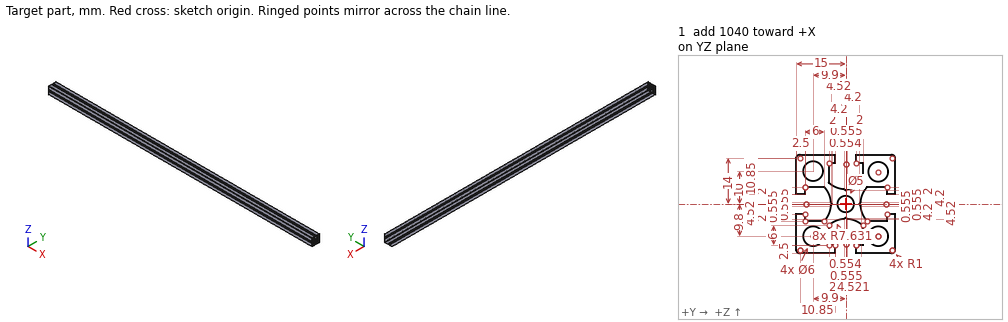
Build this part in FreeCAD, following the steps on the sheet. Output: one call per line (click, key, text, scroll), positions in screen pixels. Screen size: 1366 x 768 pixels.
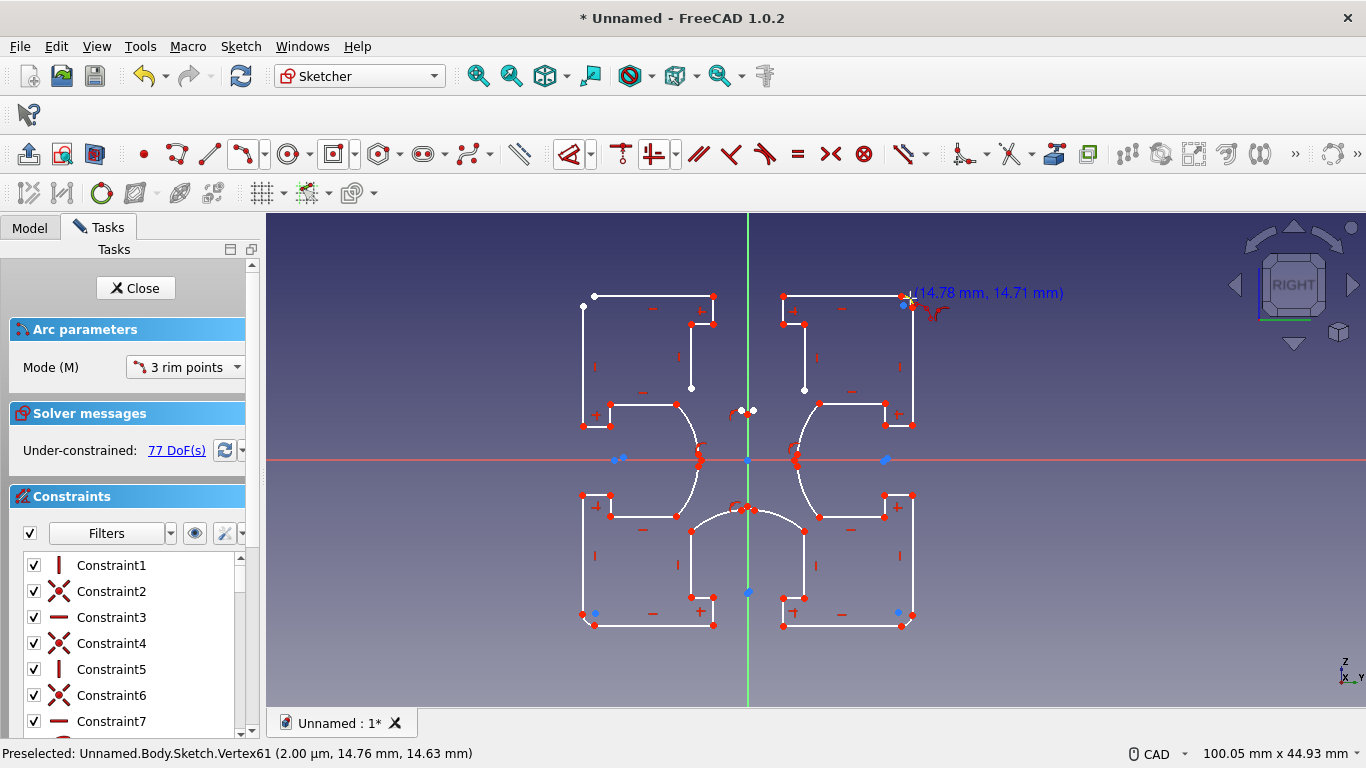
click(805, 390)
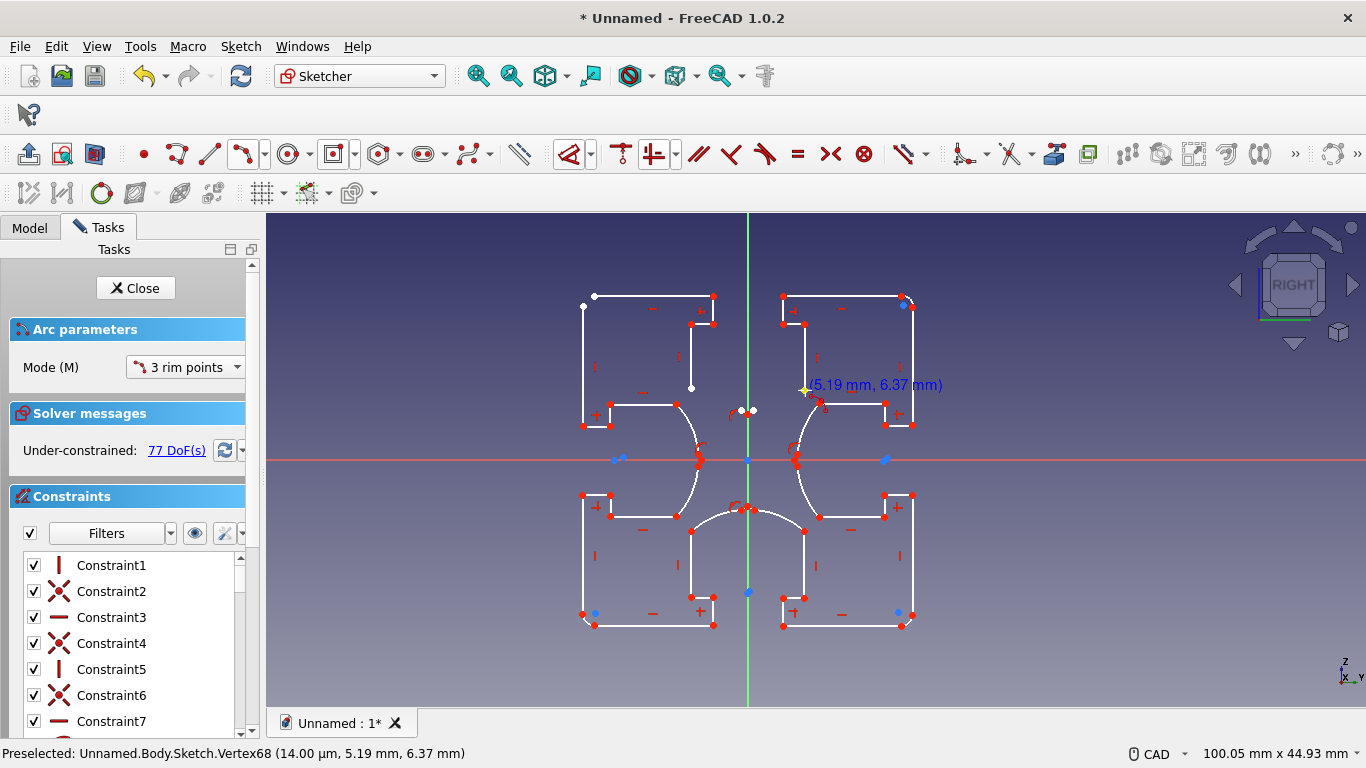
scroll(754, 410, up, 8)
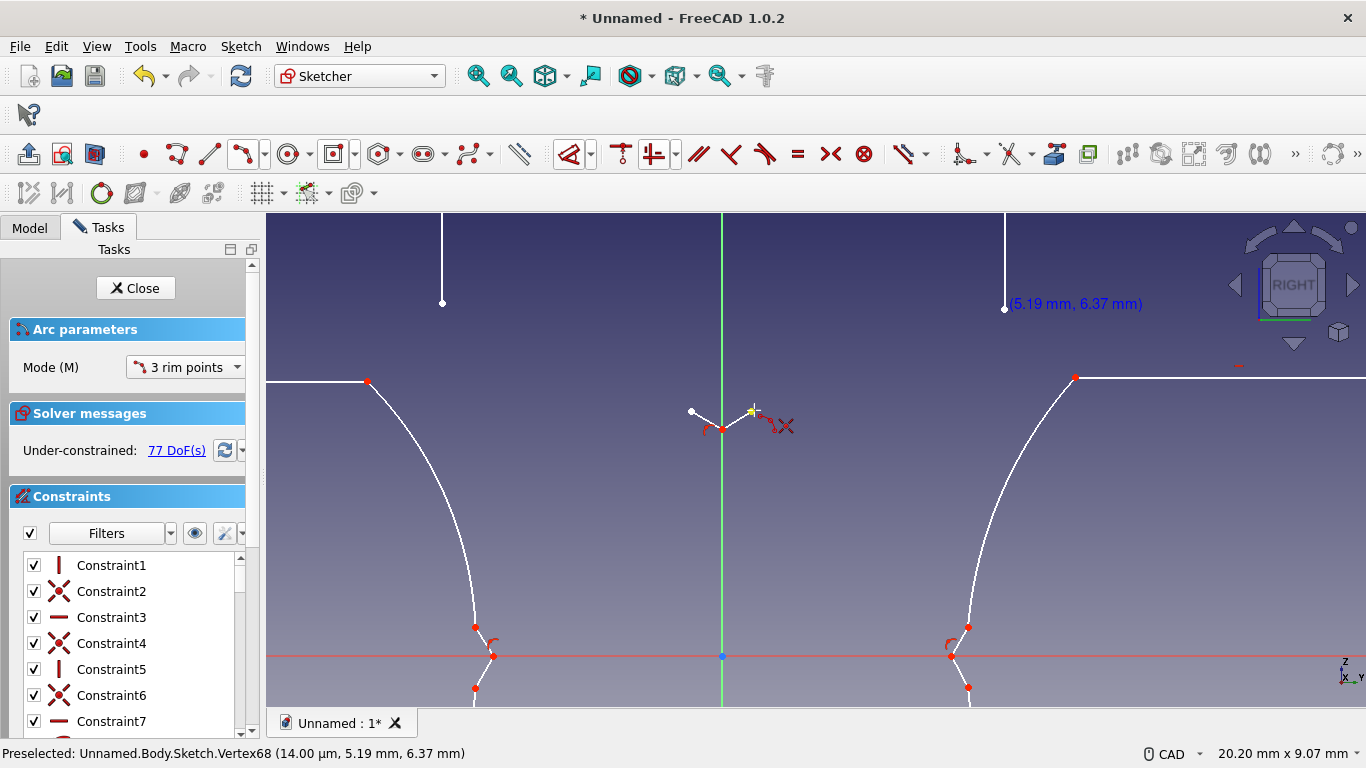
click(752, 411)
click(887, 377)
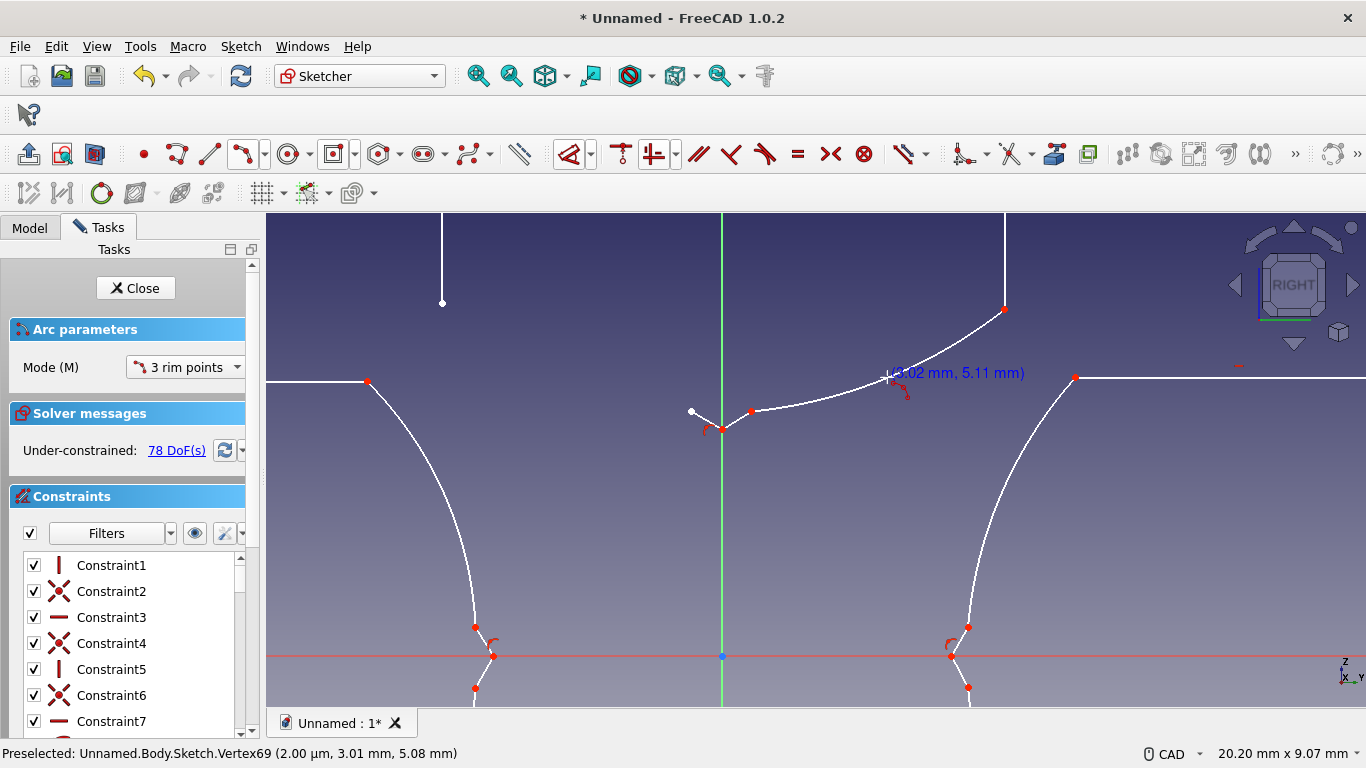
click(692, 411)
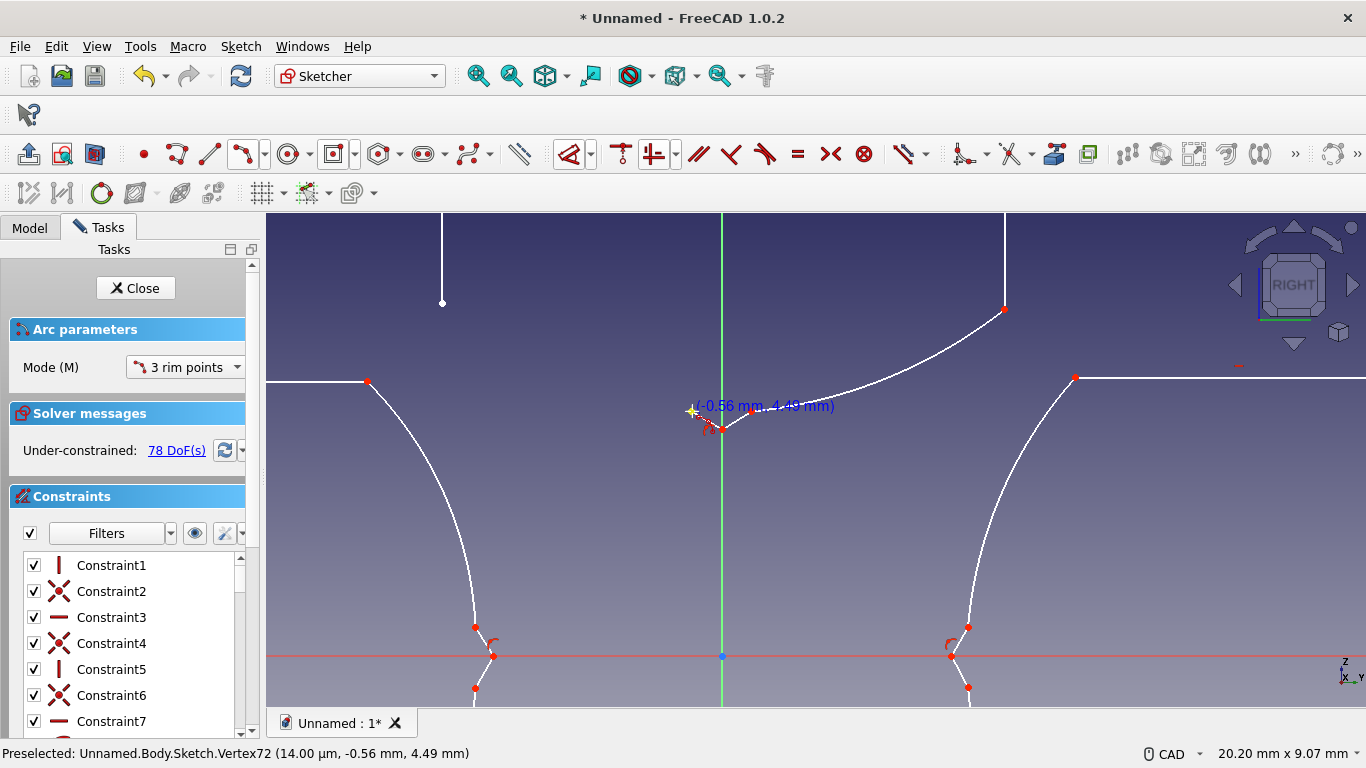
scroll(754, 410, down, 8)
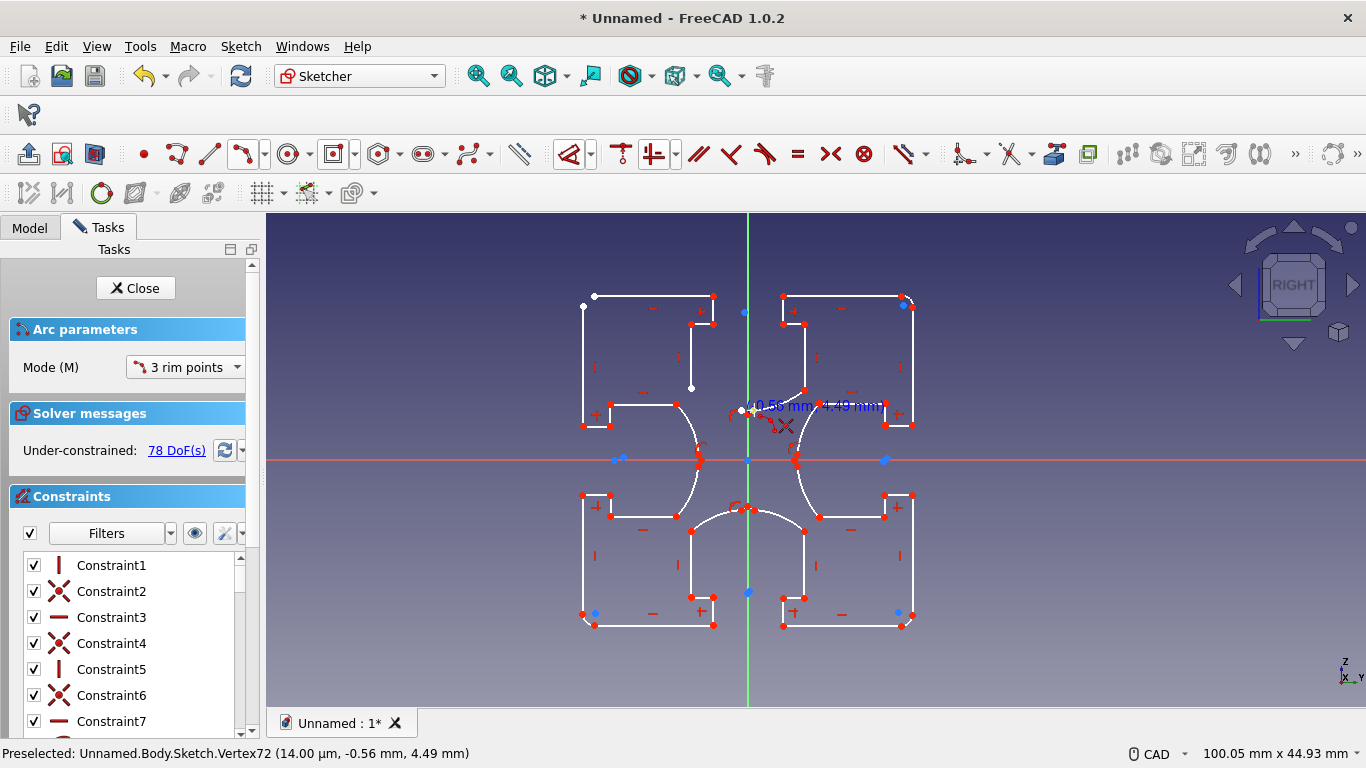
click(691, 389)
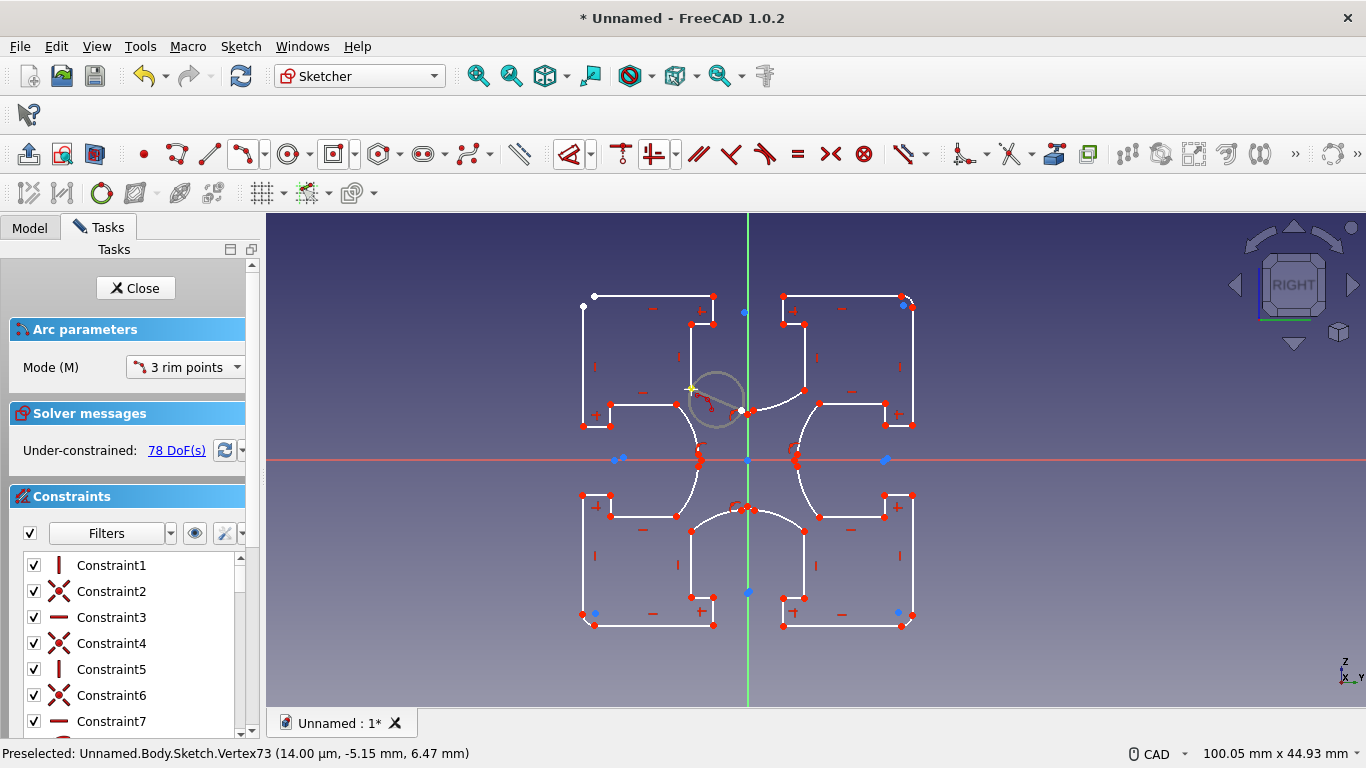
scroll(715, 404, up, 7)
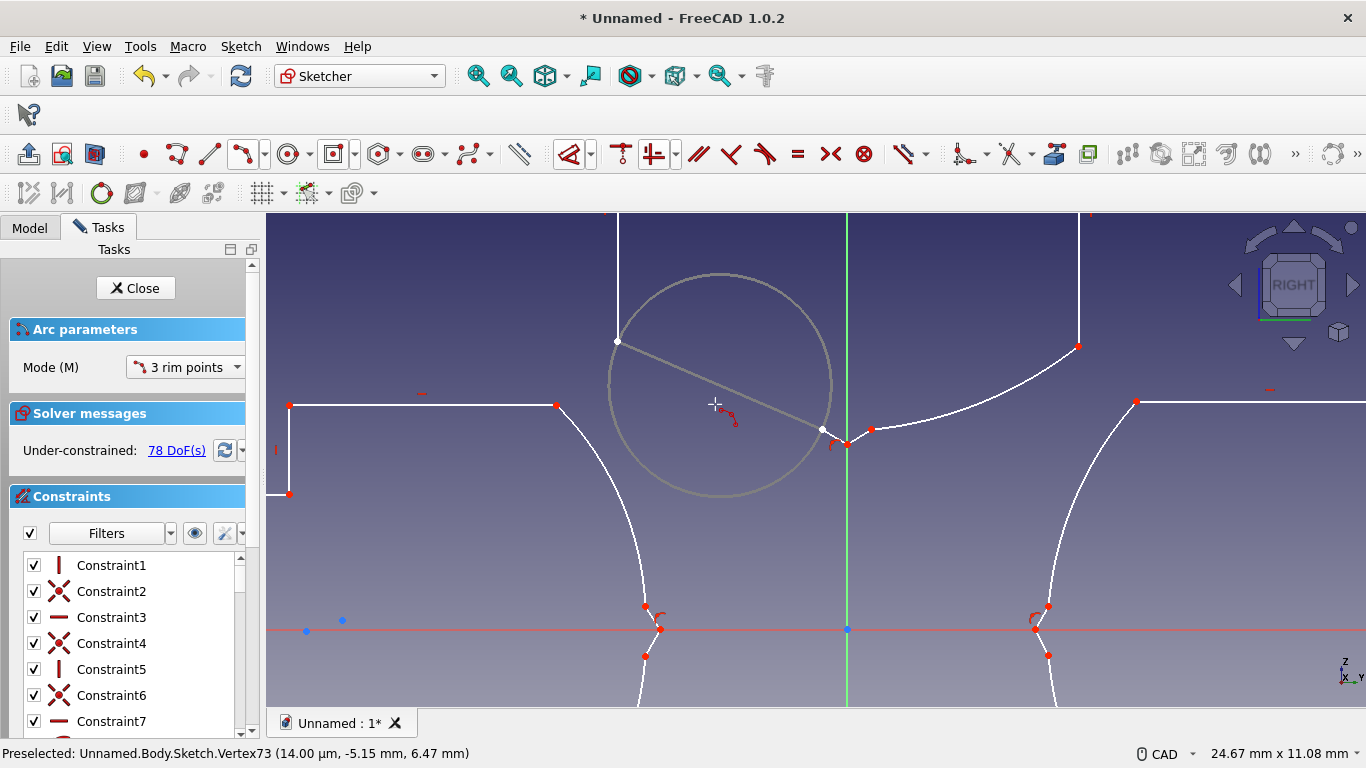
click(713, 402)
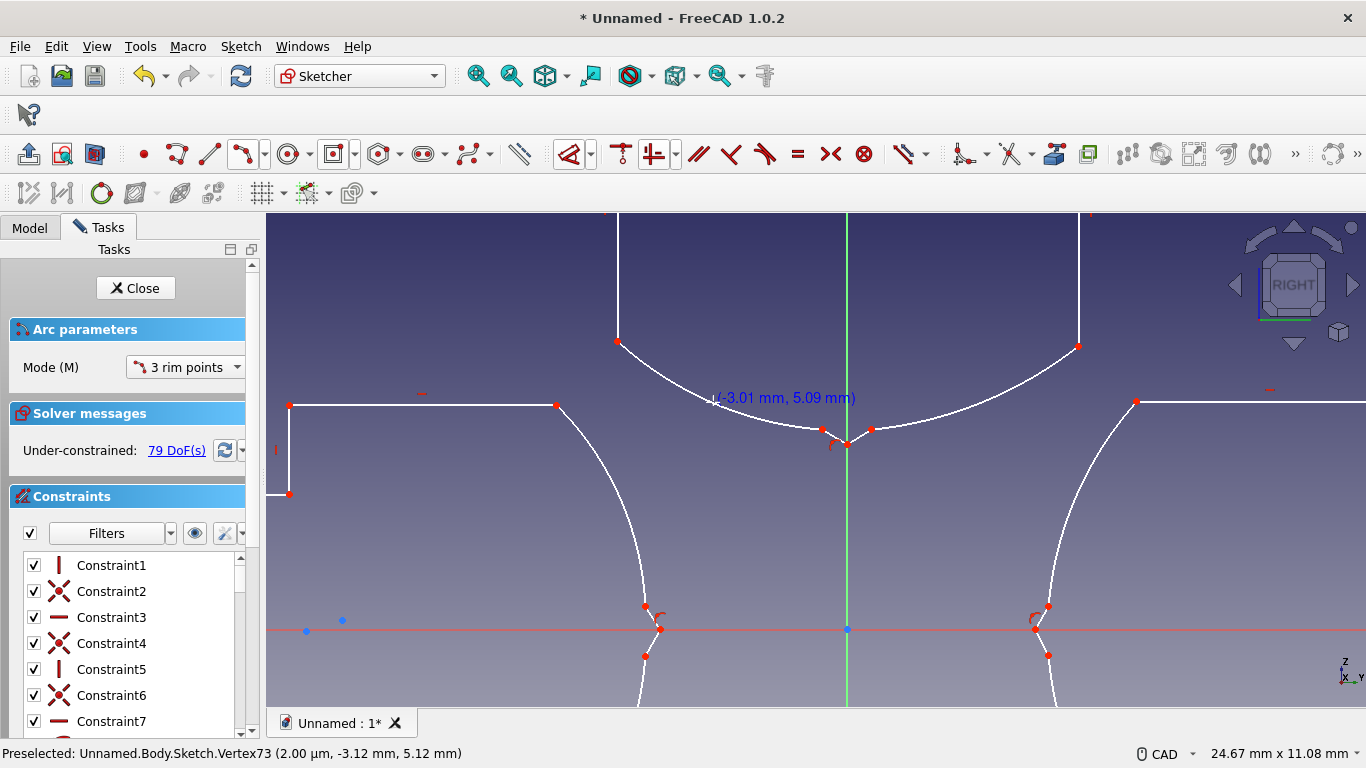
scroll(715, 404, down, 7)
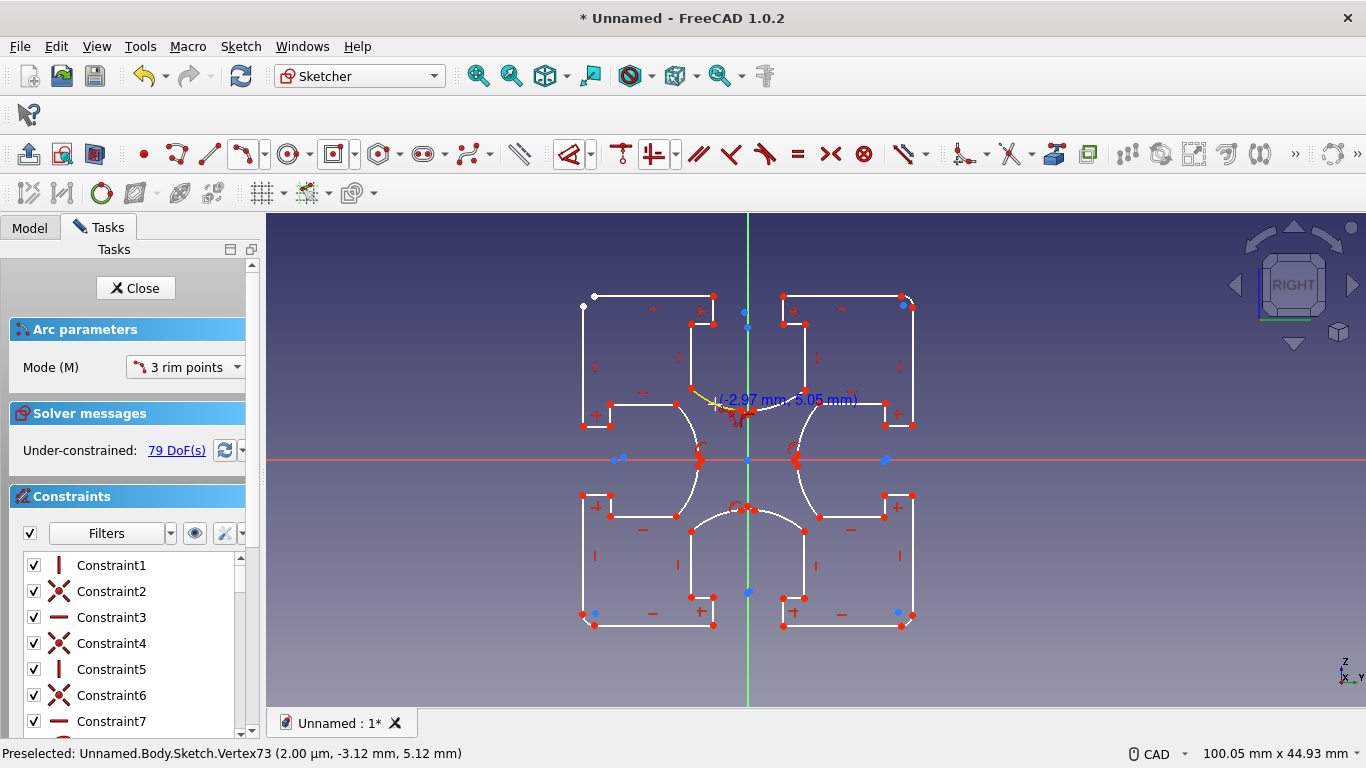
click(594, 296)
click(583, 307)